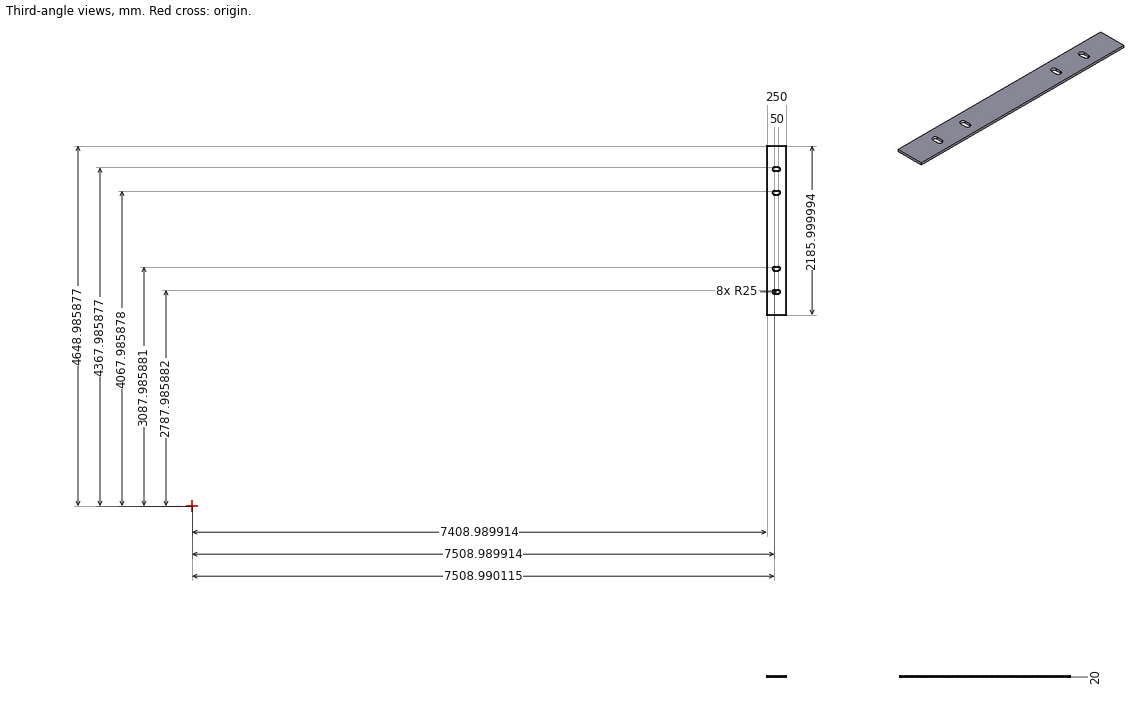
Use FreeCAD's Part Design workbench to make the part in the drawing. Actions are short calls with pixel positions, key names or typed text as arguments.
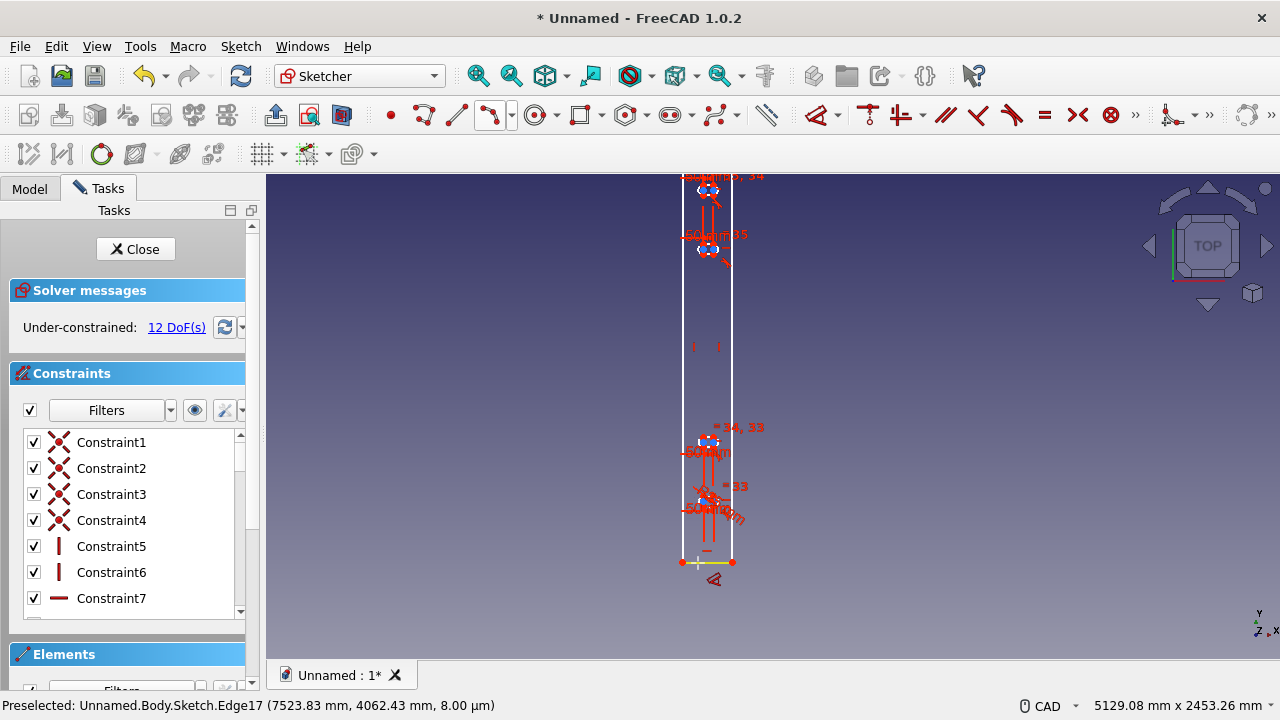
click(698, 563)
click(707, 597)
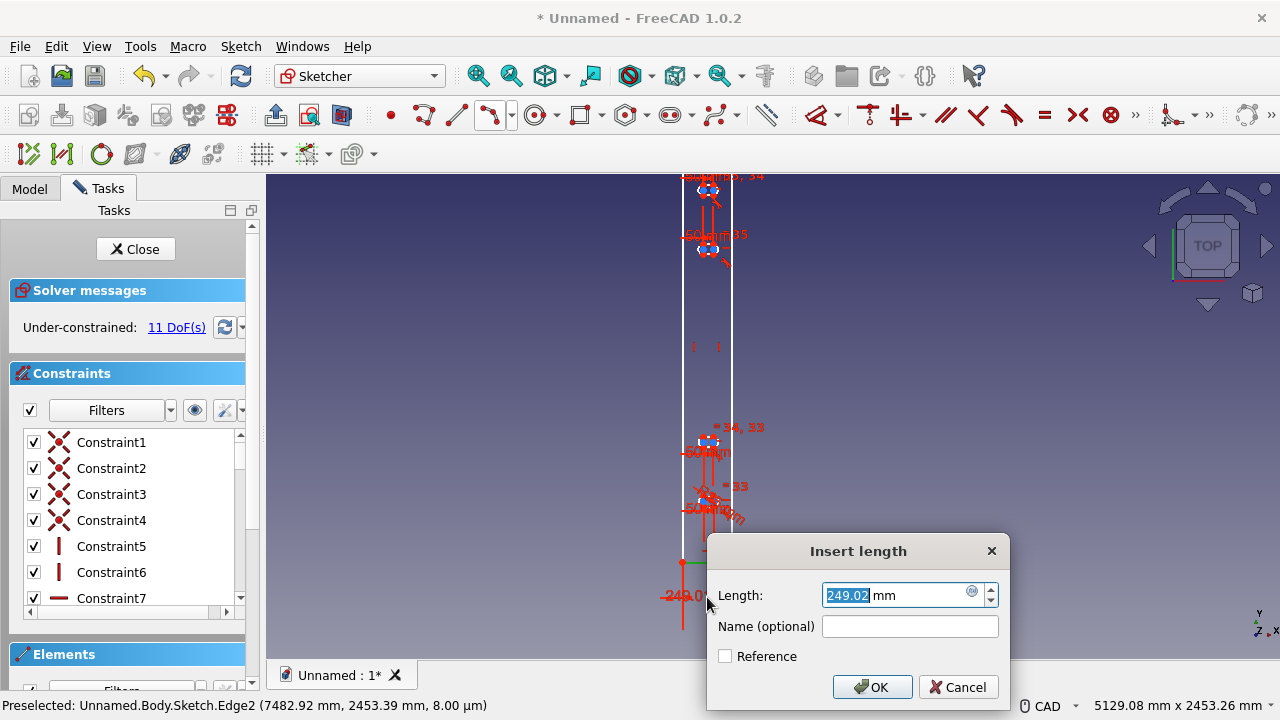
text(250)
key(Return)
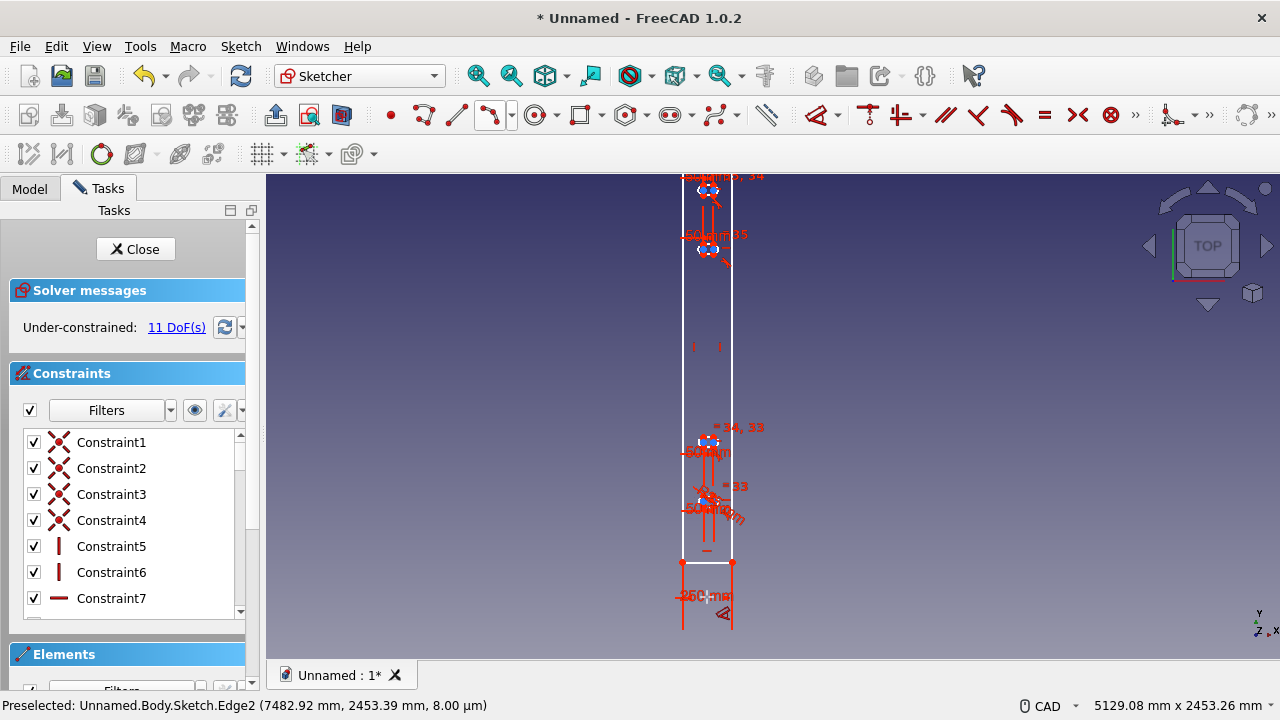
click(683, 260)
click(649, 382)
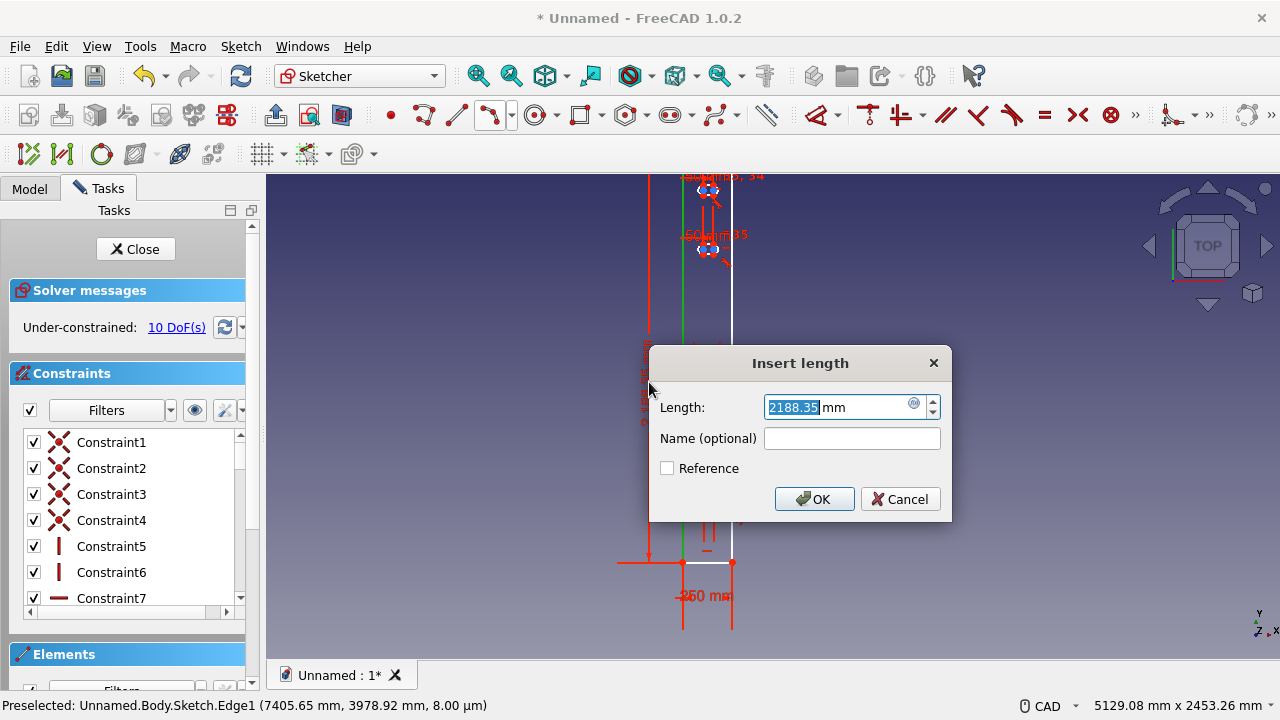
text(2185.999994)
key(Return)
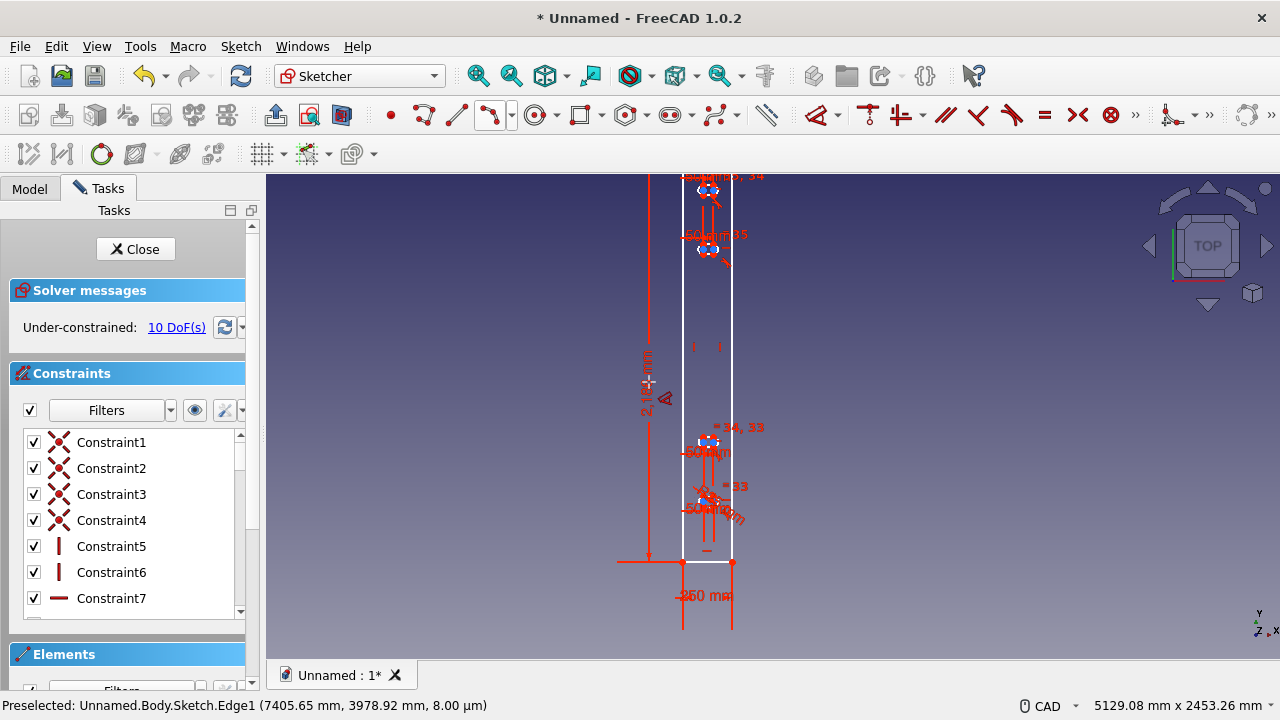
scroll(697, 563, down, 2)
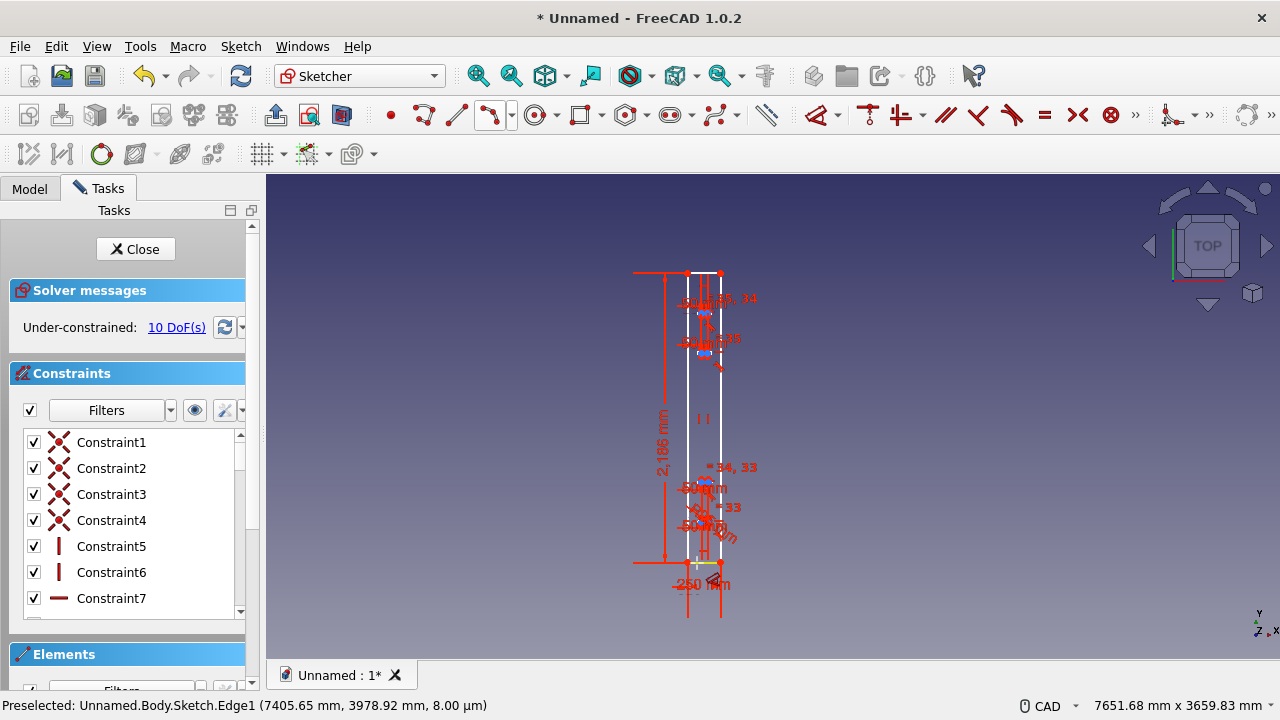
click(688, 273)
click(491, 239)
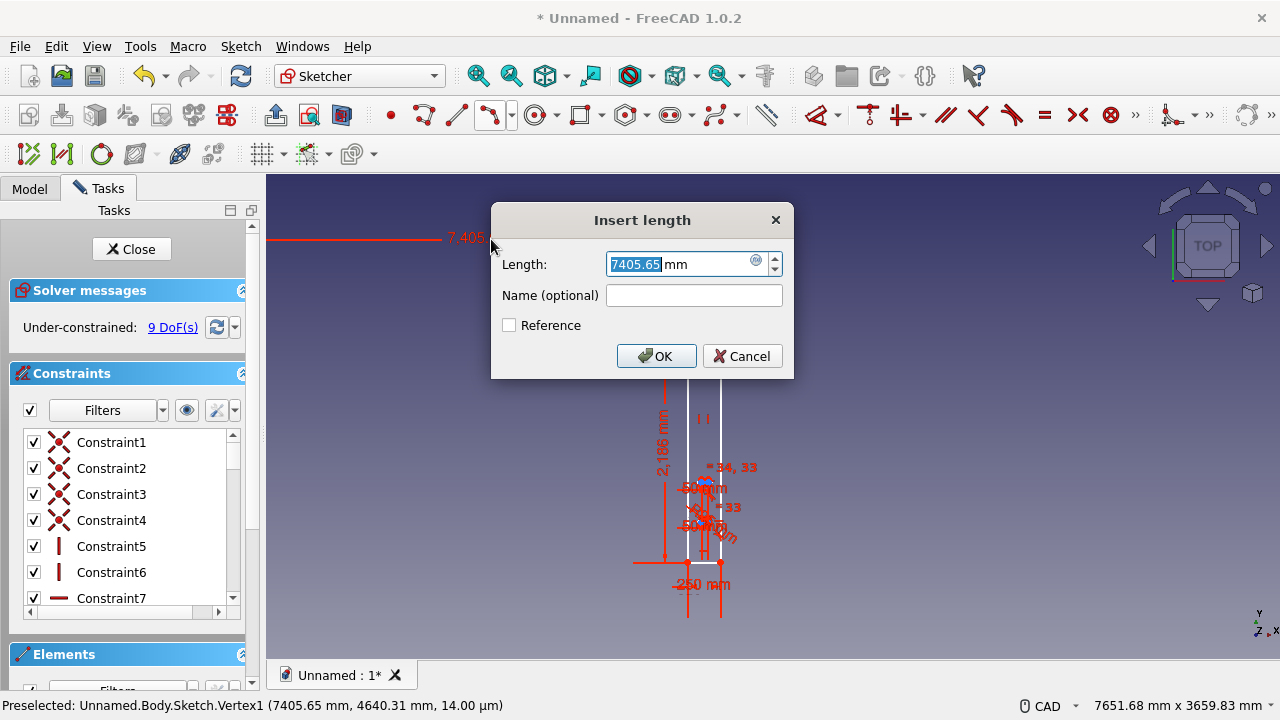
text(7408.989914)
key(Return)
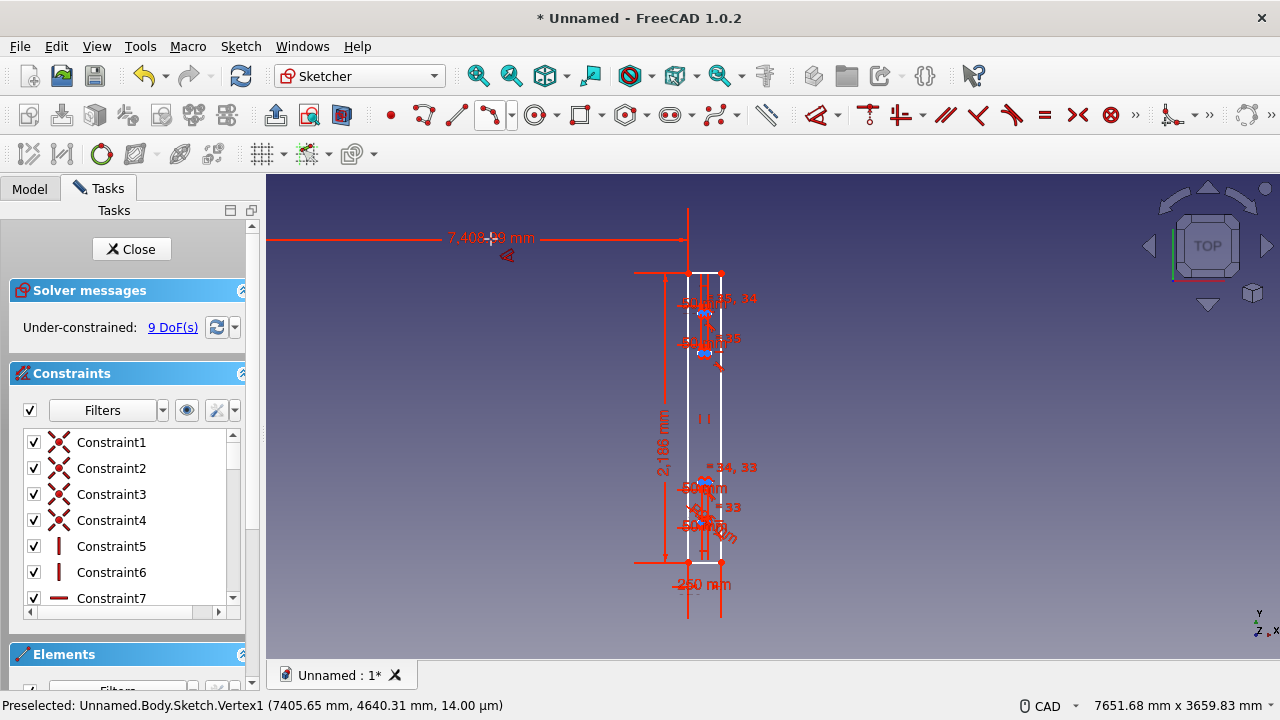
click(688, 273)
click(746, 452)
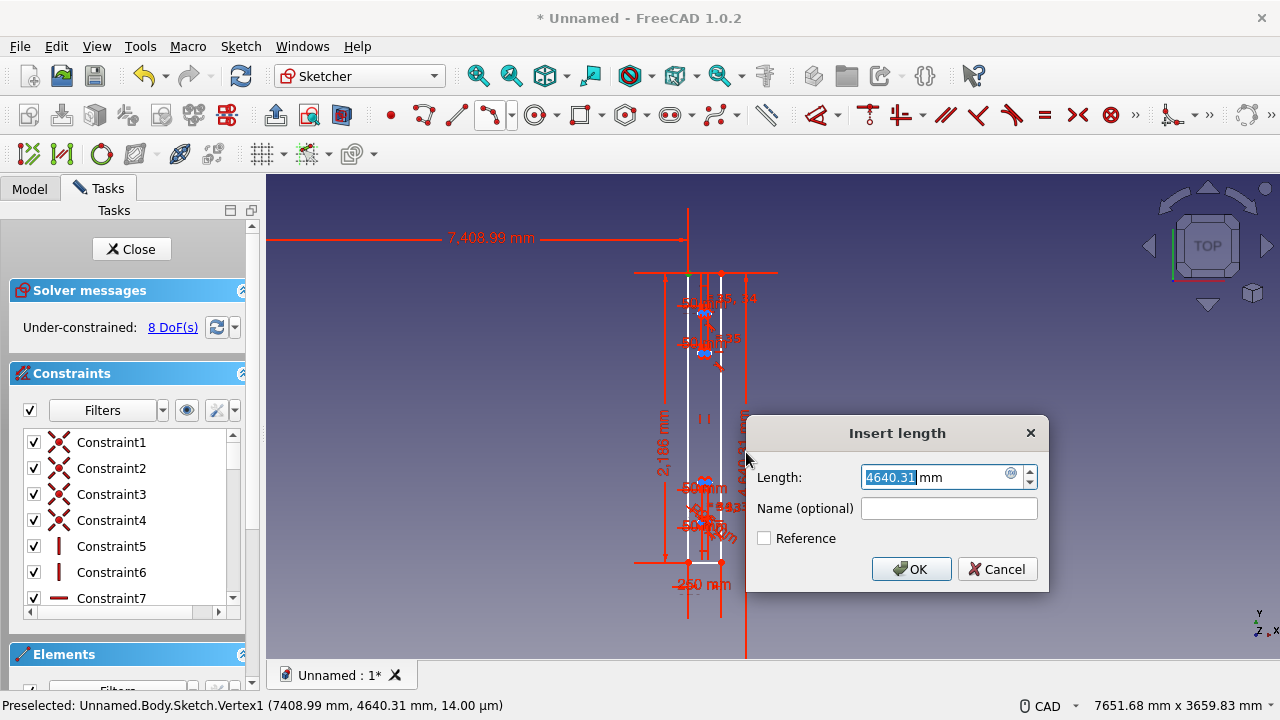
text(4648.985877)
key(Return)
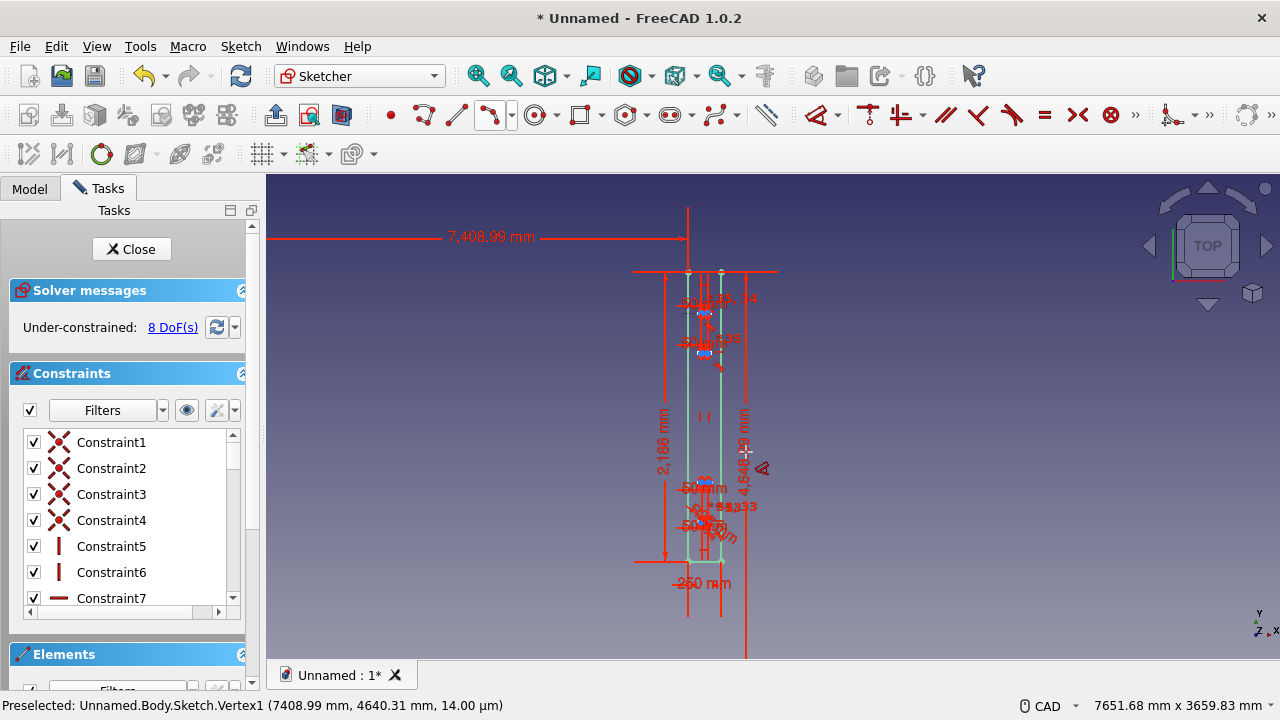
scroll(702, 519, up, 7)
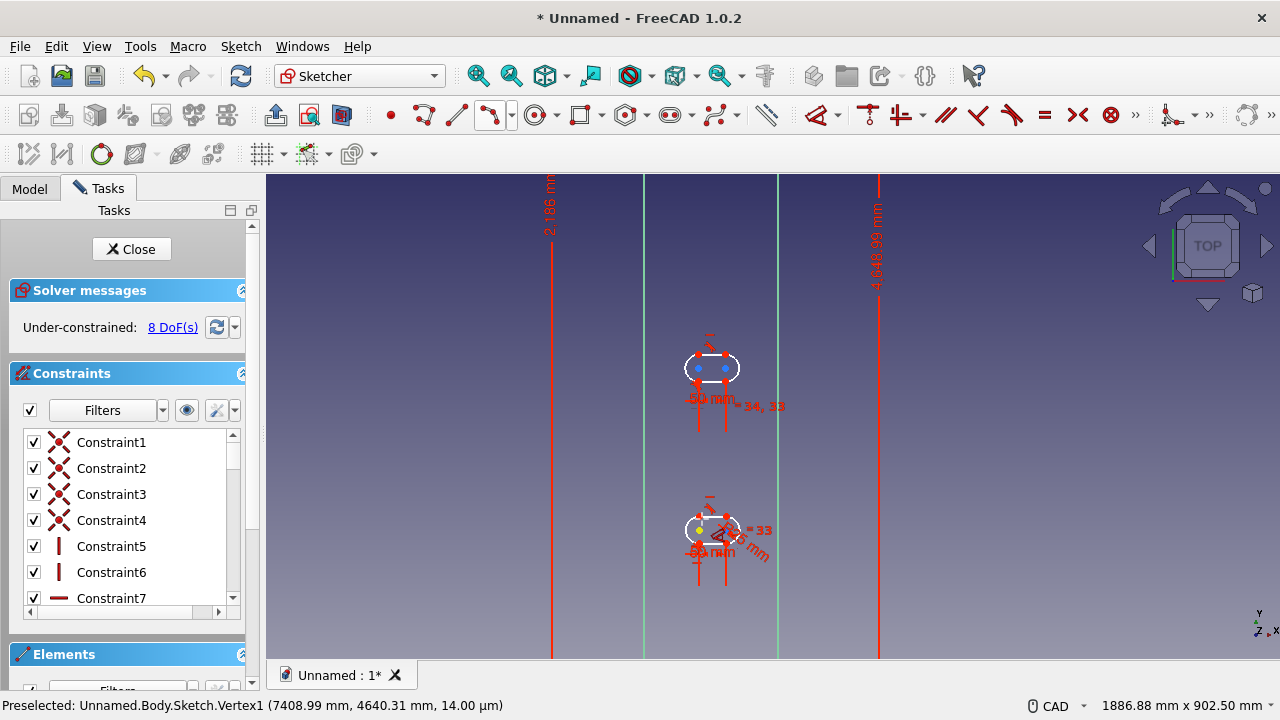
click(699, 517)
click(497, 483)